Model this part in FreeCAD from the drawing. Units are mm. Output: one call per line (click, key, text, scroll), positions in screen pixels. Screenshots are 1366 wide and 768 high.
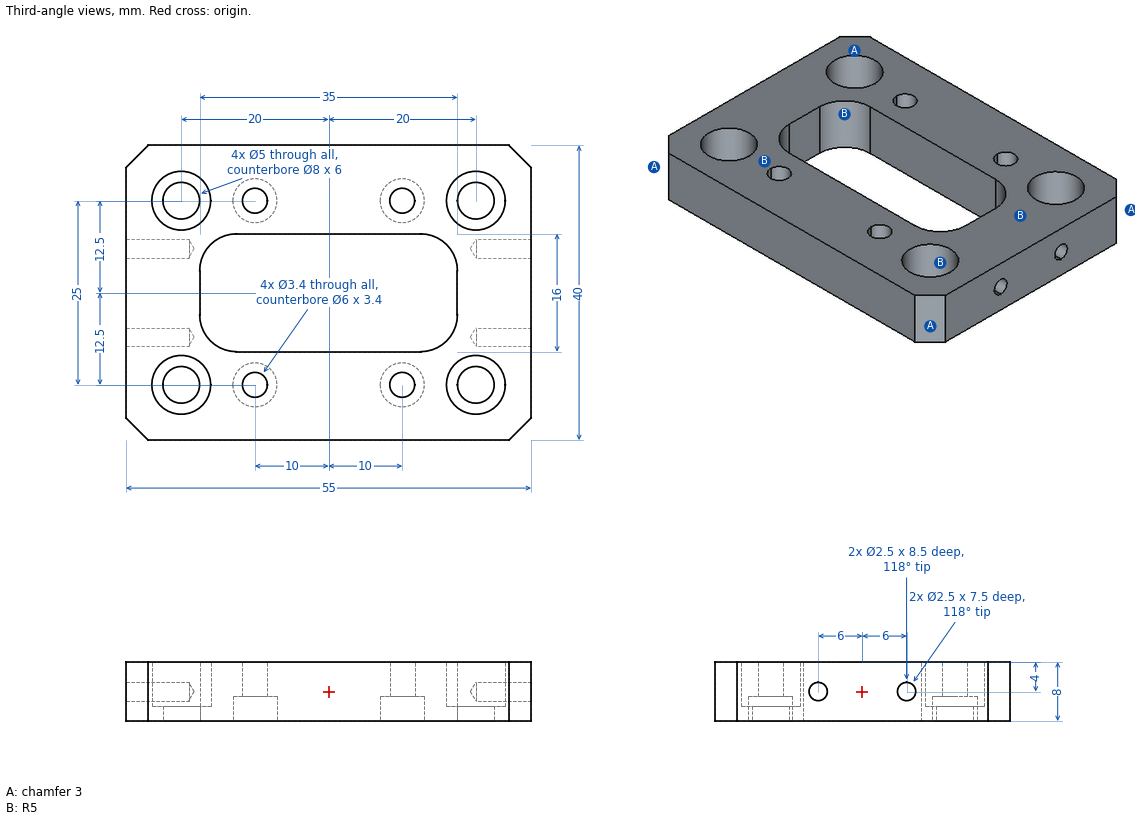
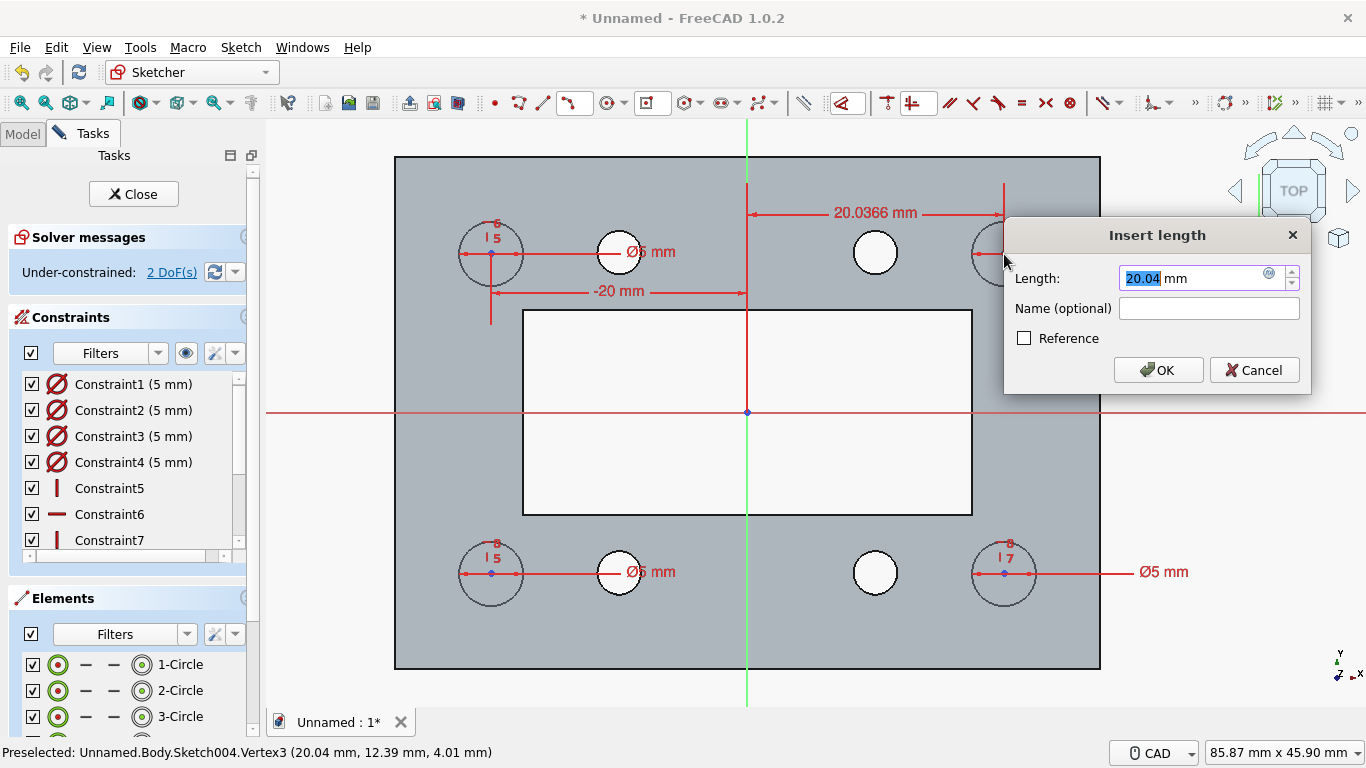
text(20)
key(Return)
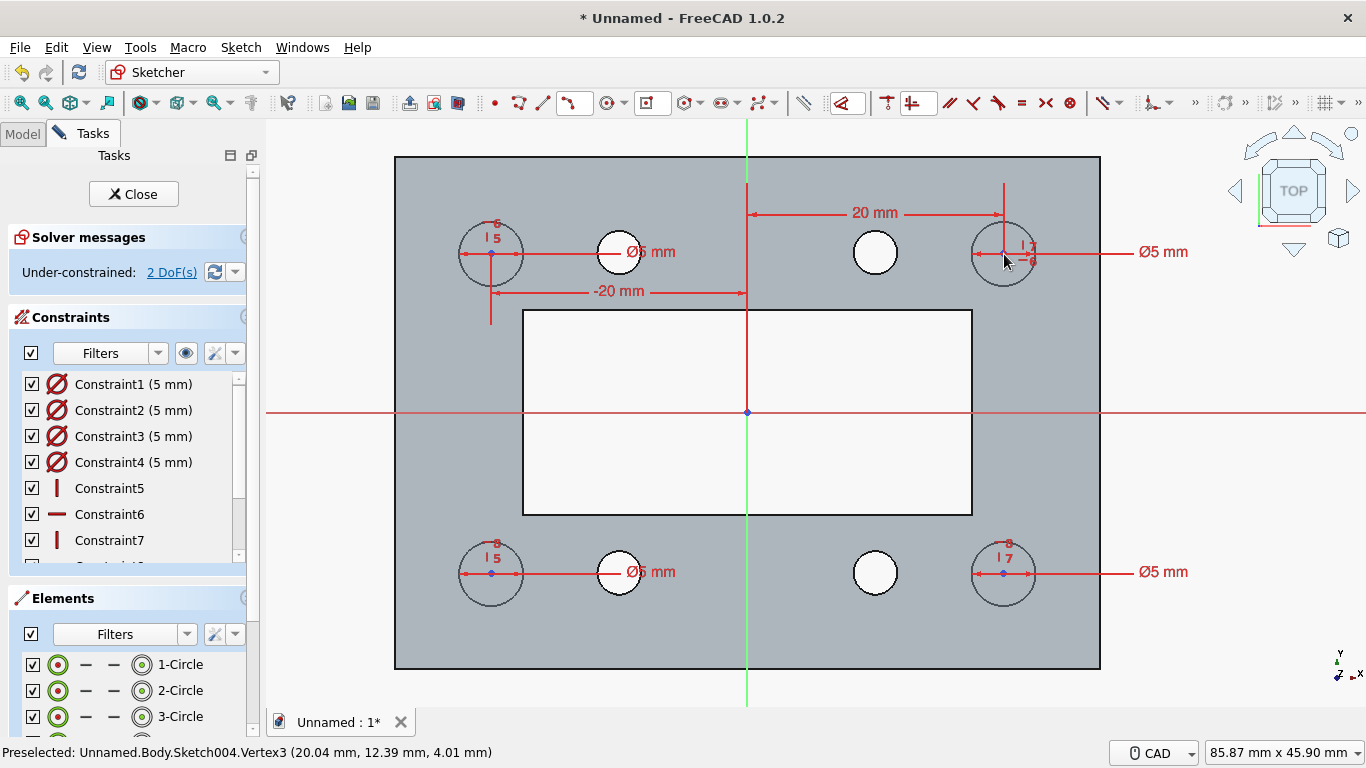
click(491, 254)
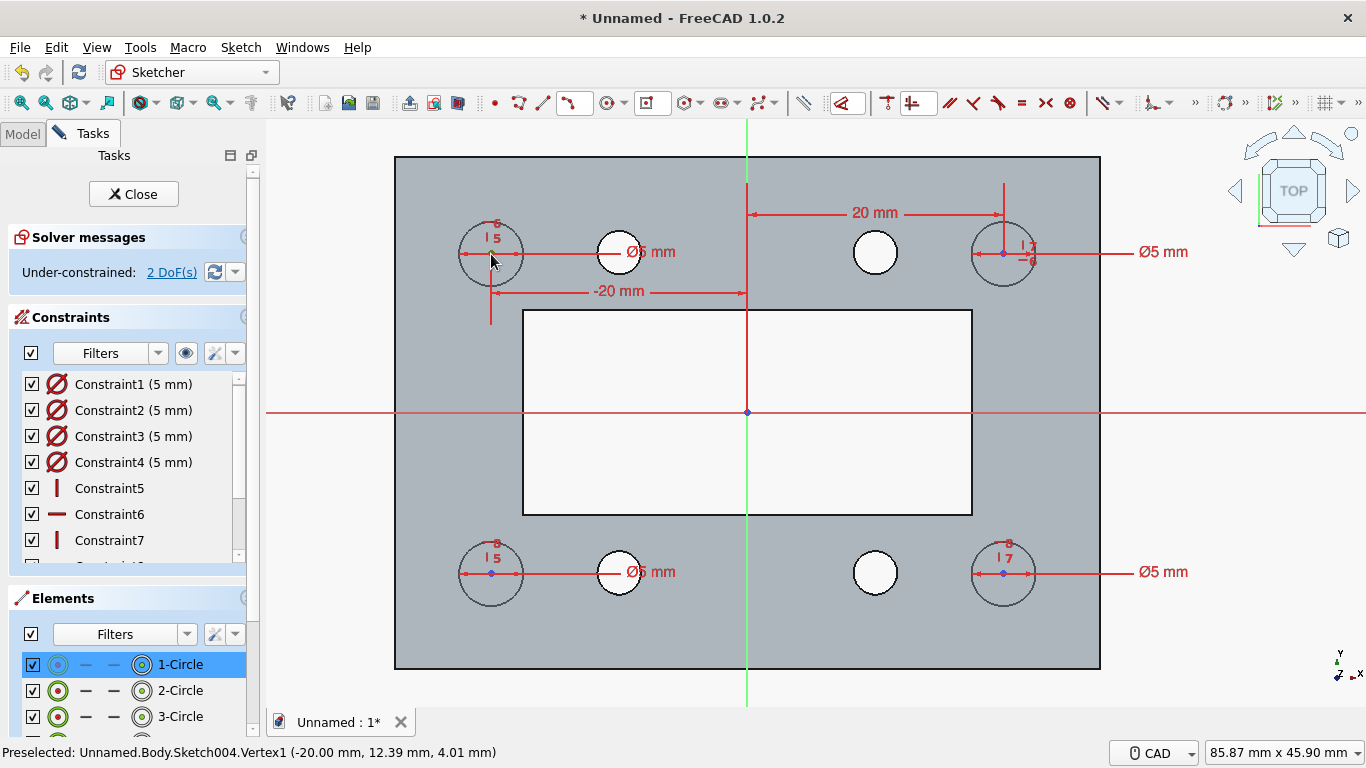
click(491, 574)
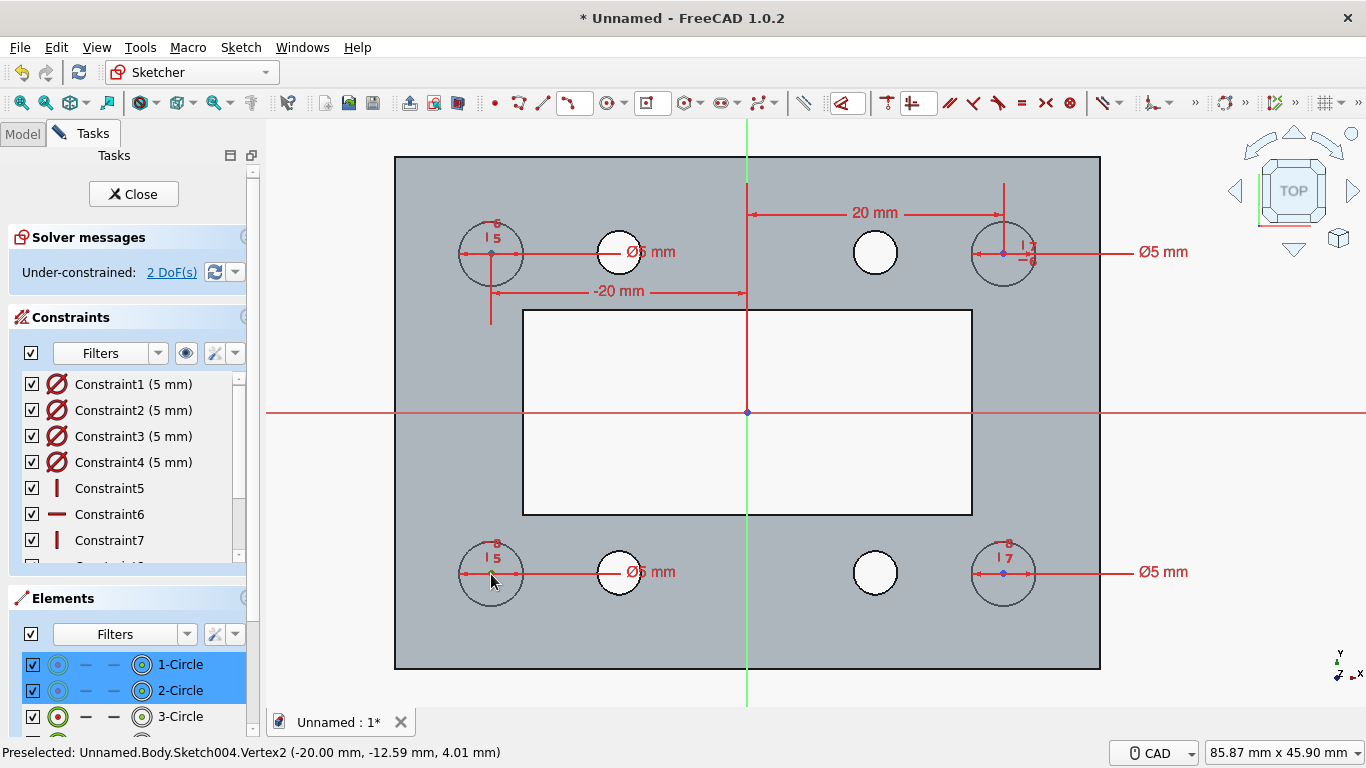
key(i)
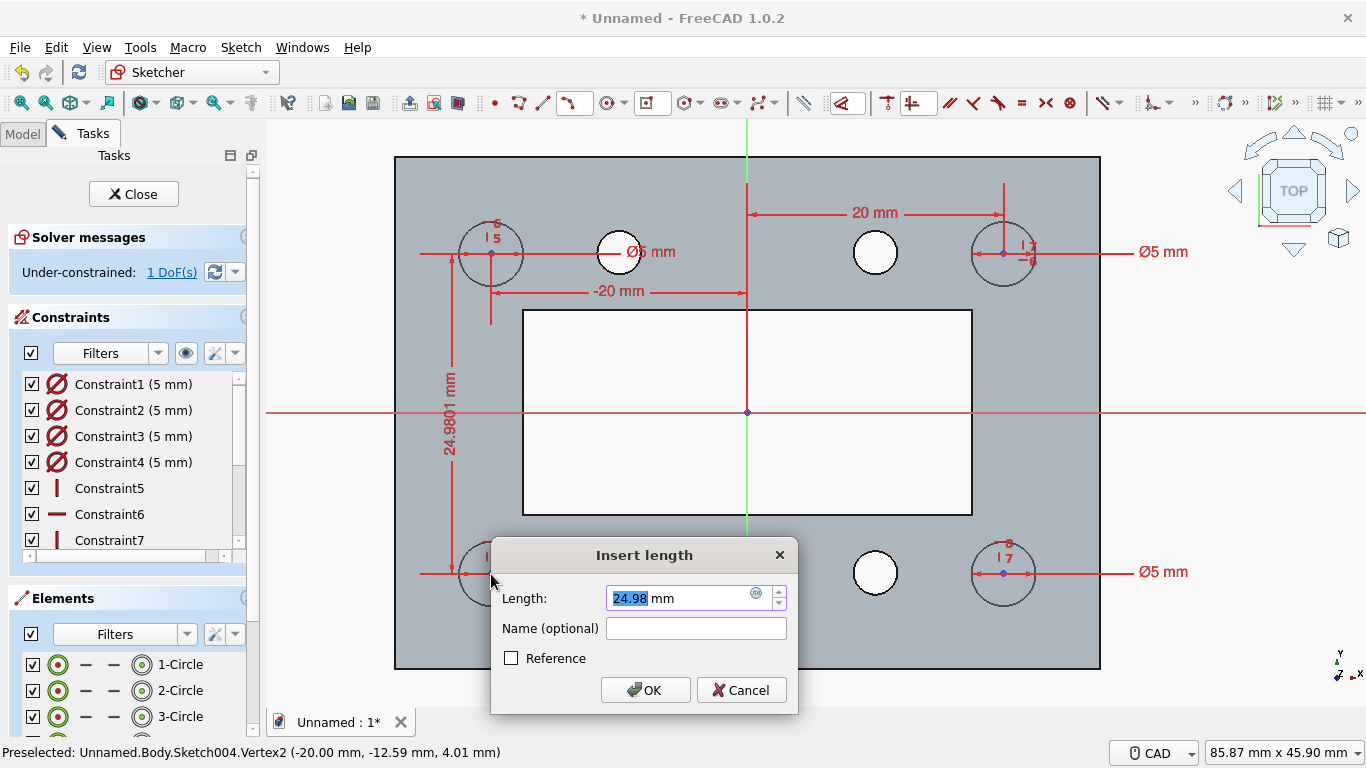
text(25)
key(Return)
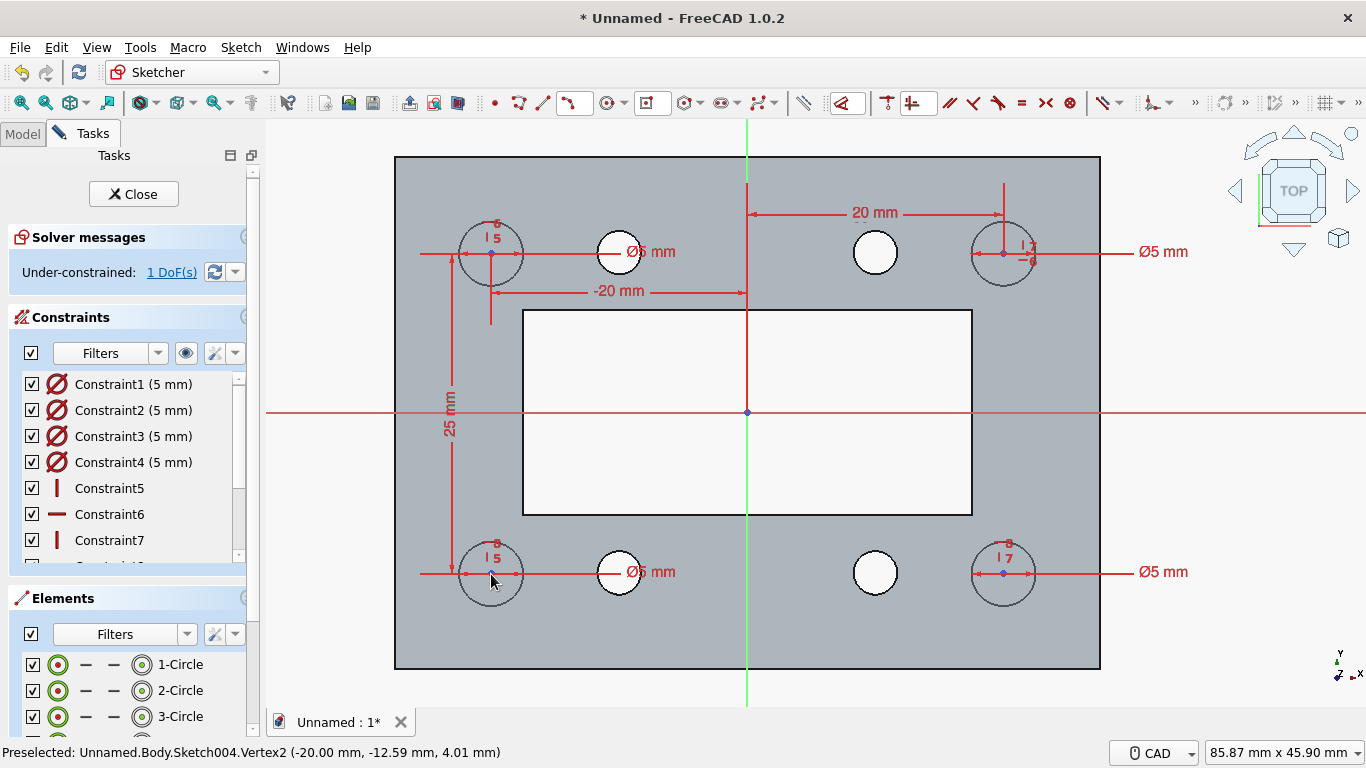
click(491, 254)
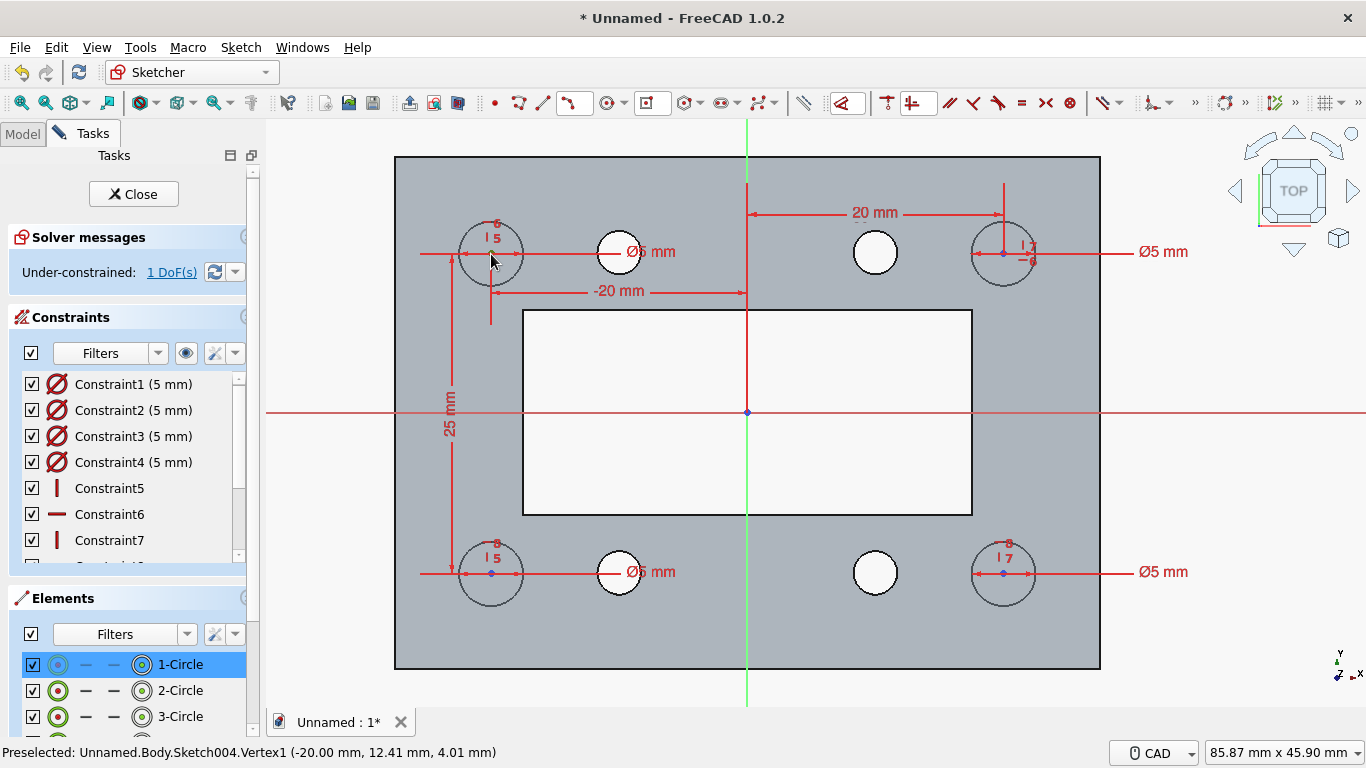
key(i)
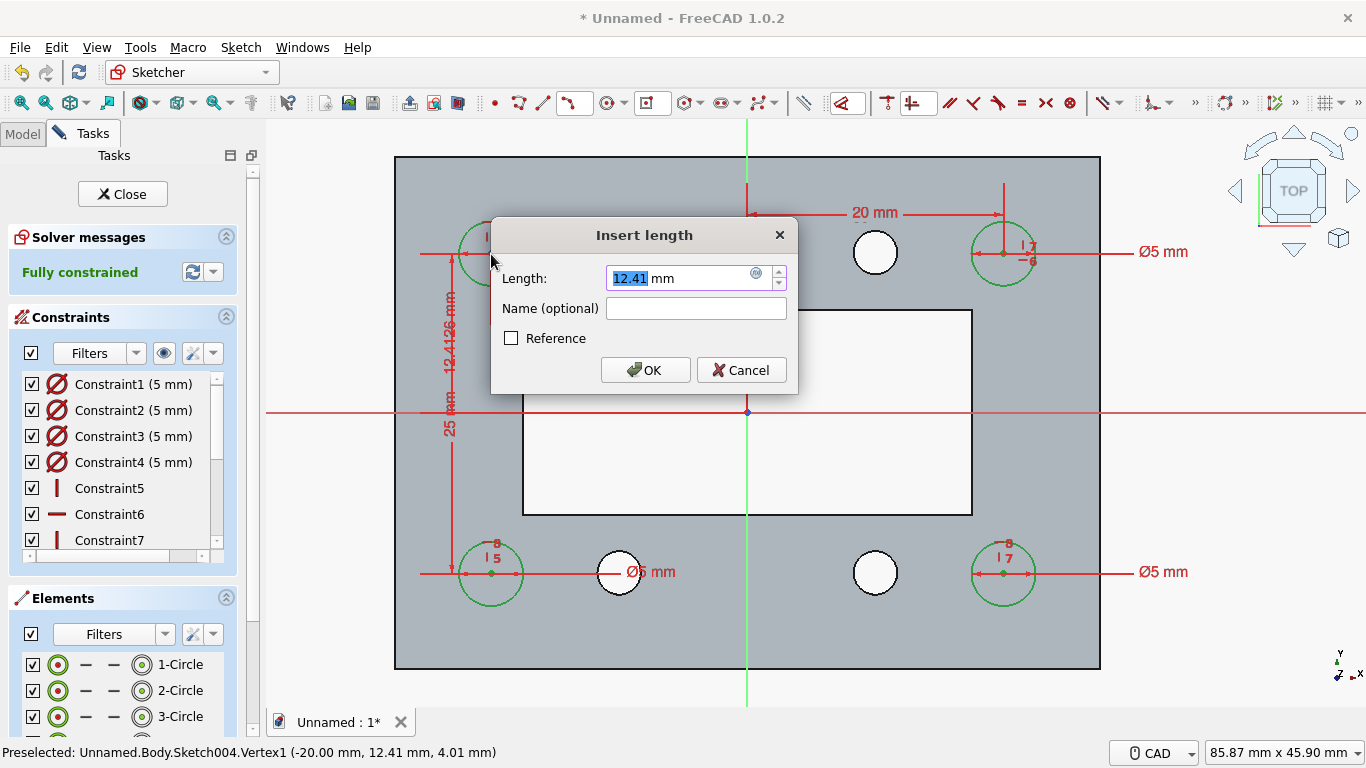
text(12.5)
key(Return)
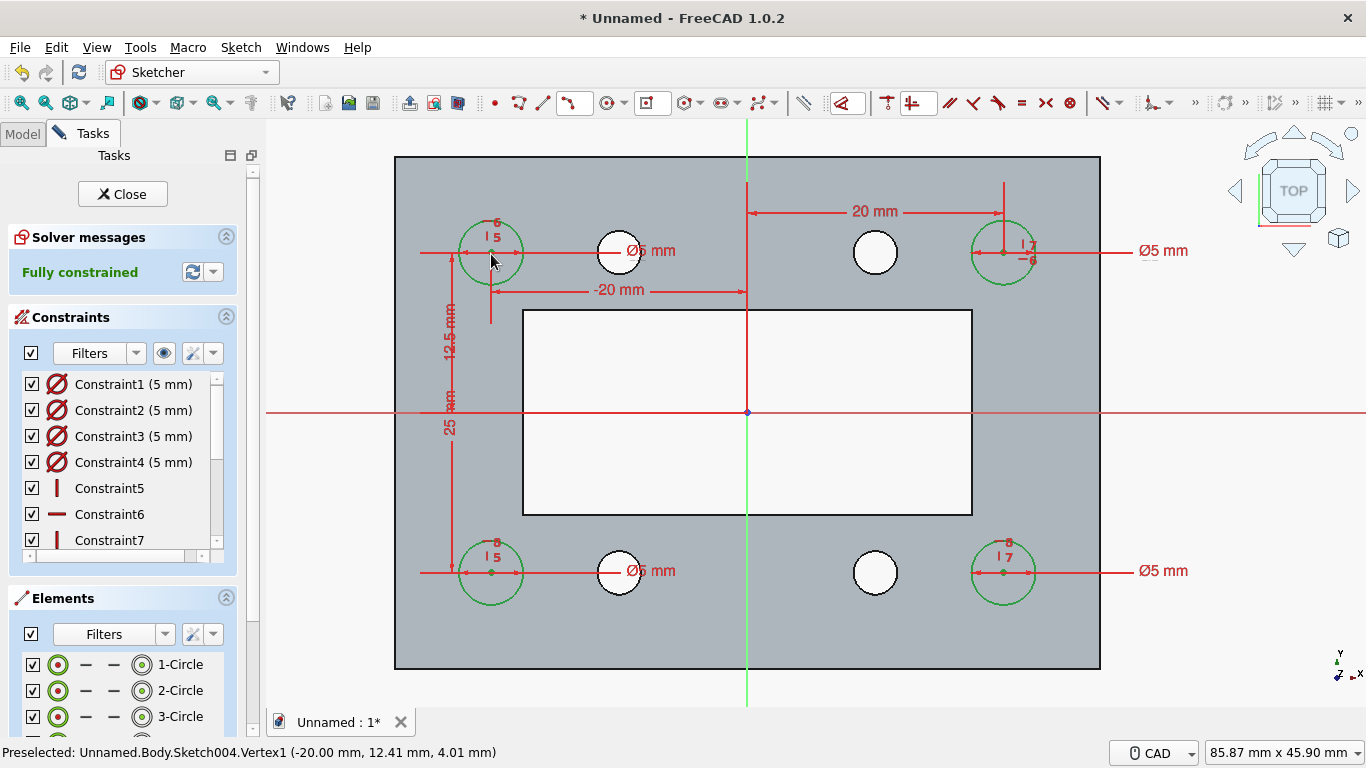
click(123, 194)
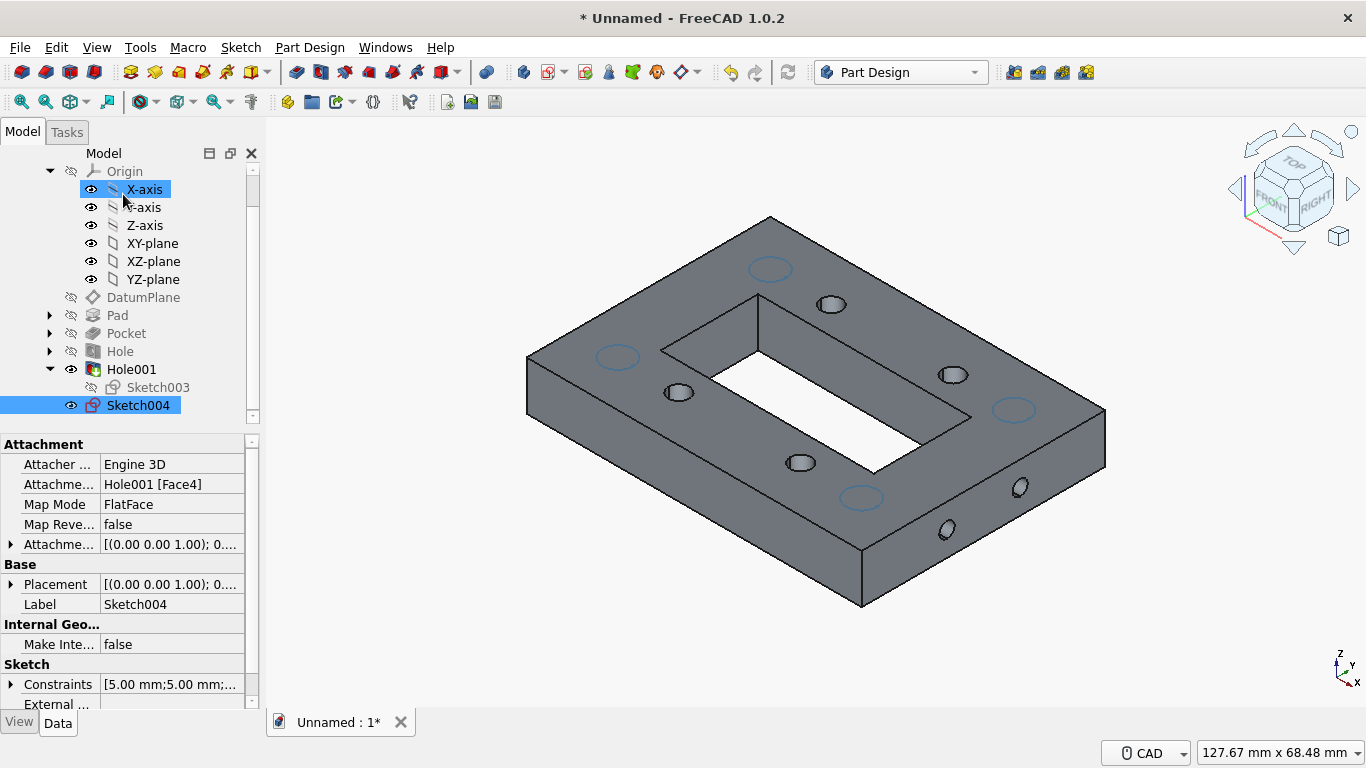
click(322, 72)